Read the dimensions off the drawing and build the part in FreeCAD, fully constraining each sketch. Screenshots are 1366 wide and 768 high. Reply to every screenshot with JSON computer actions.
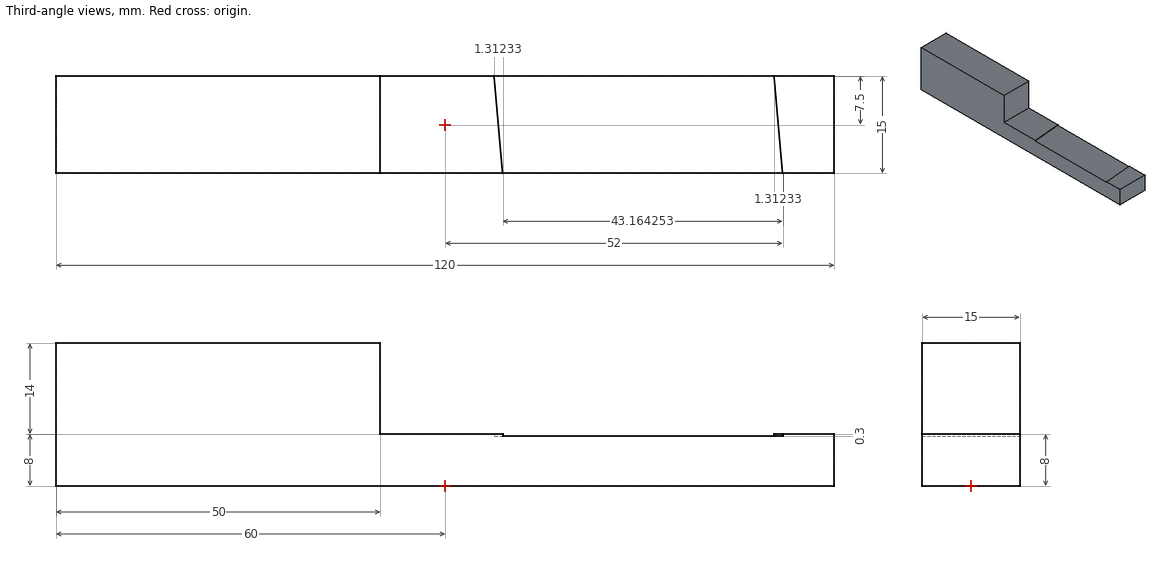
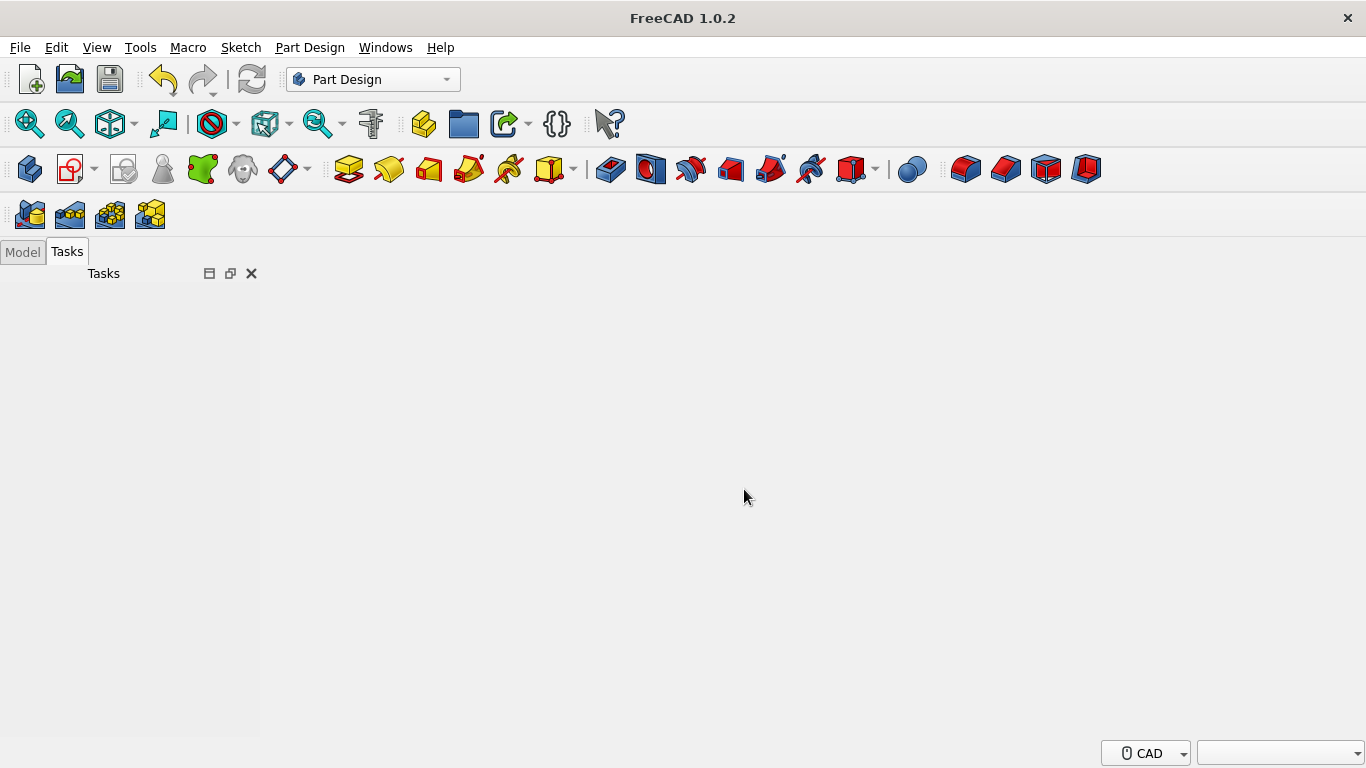
{"action": "left_click", "coordinate": [30, 80]}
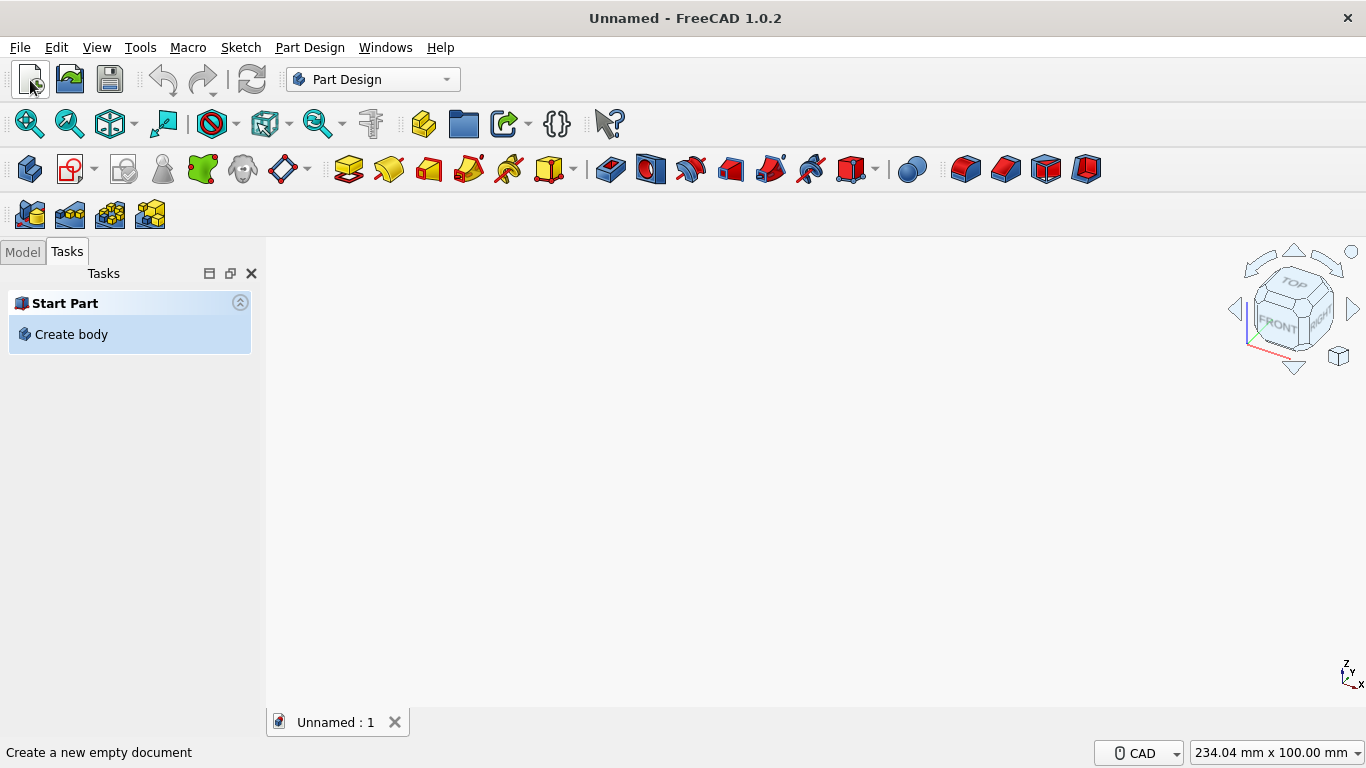
{"action": "left_click", "coordinate": [70, 170]}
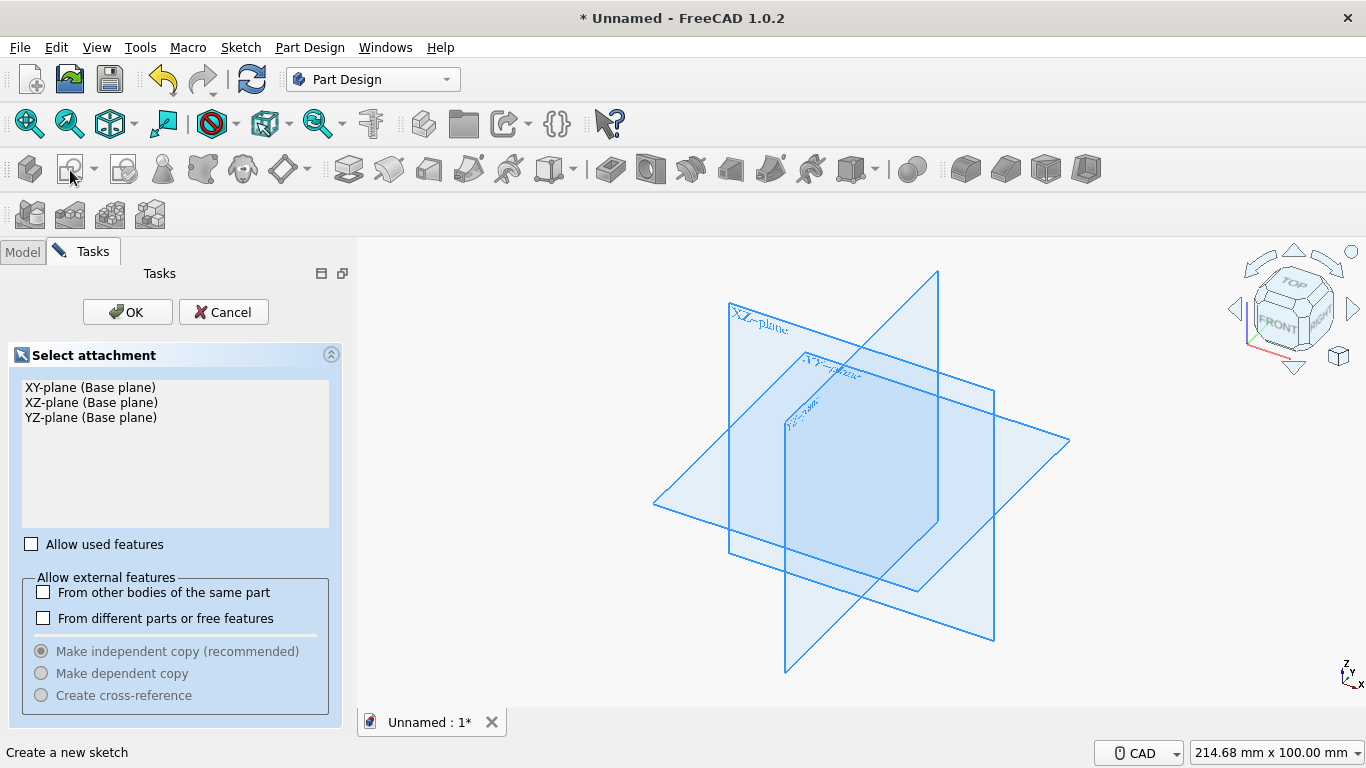
{"action": "left_click", "coordinate": [82, 388]}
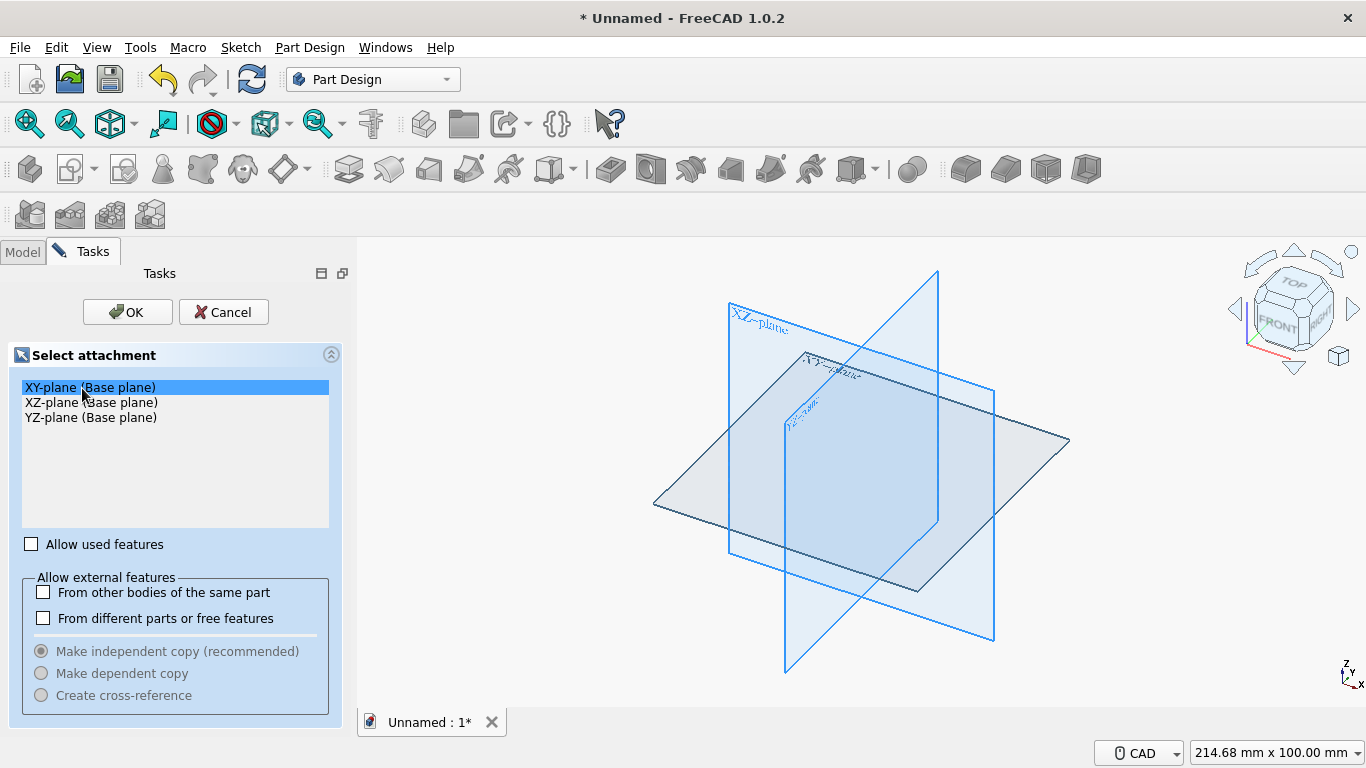
{"action": "left_click", "coordinate": [128, 312]}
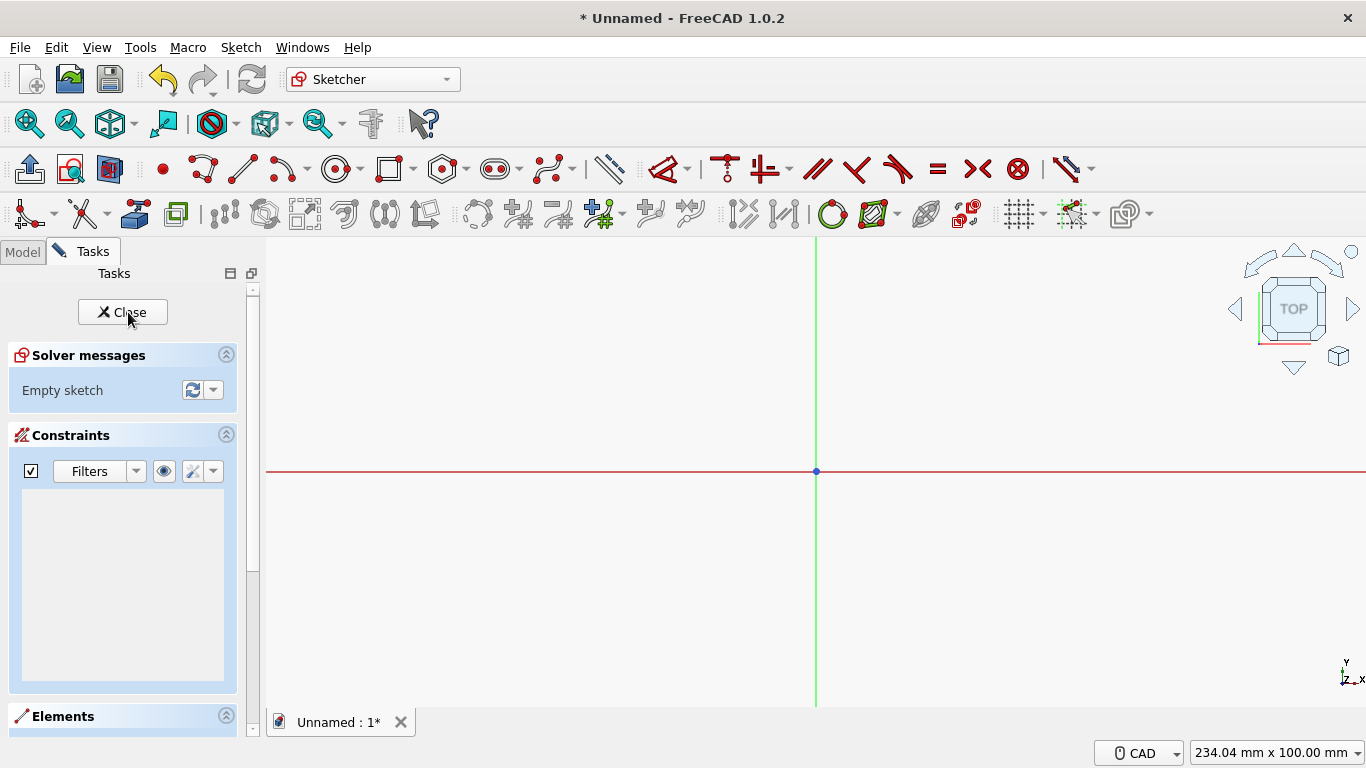
{"action": "left_click", "coordinate": [416, 170]}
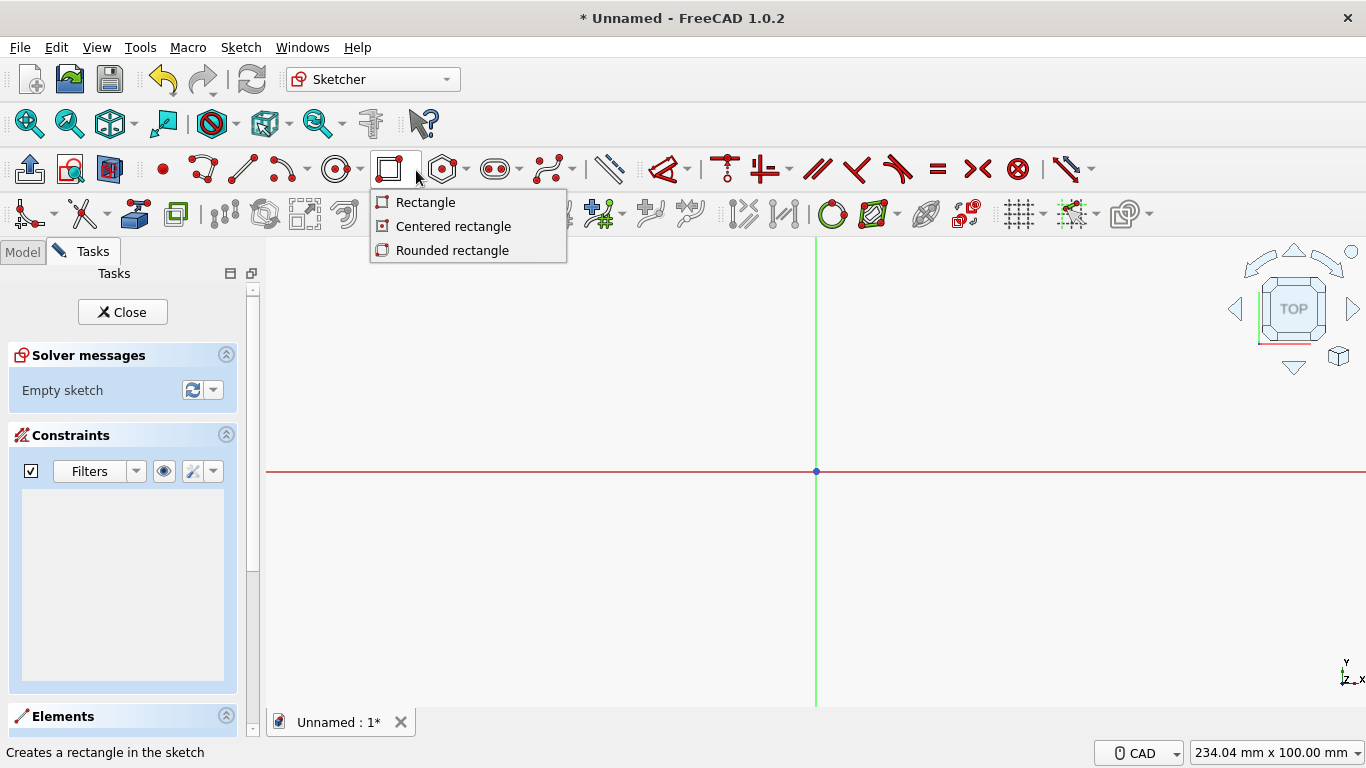
{"action": "left_click", "coordinate": [468, 226]}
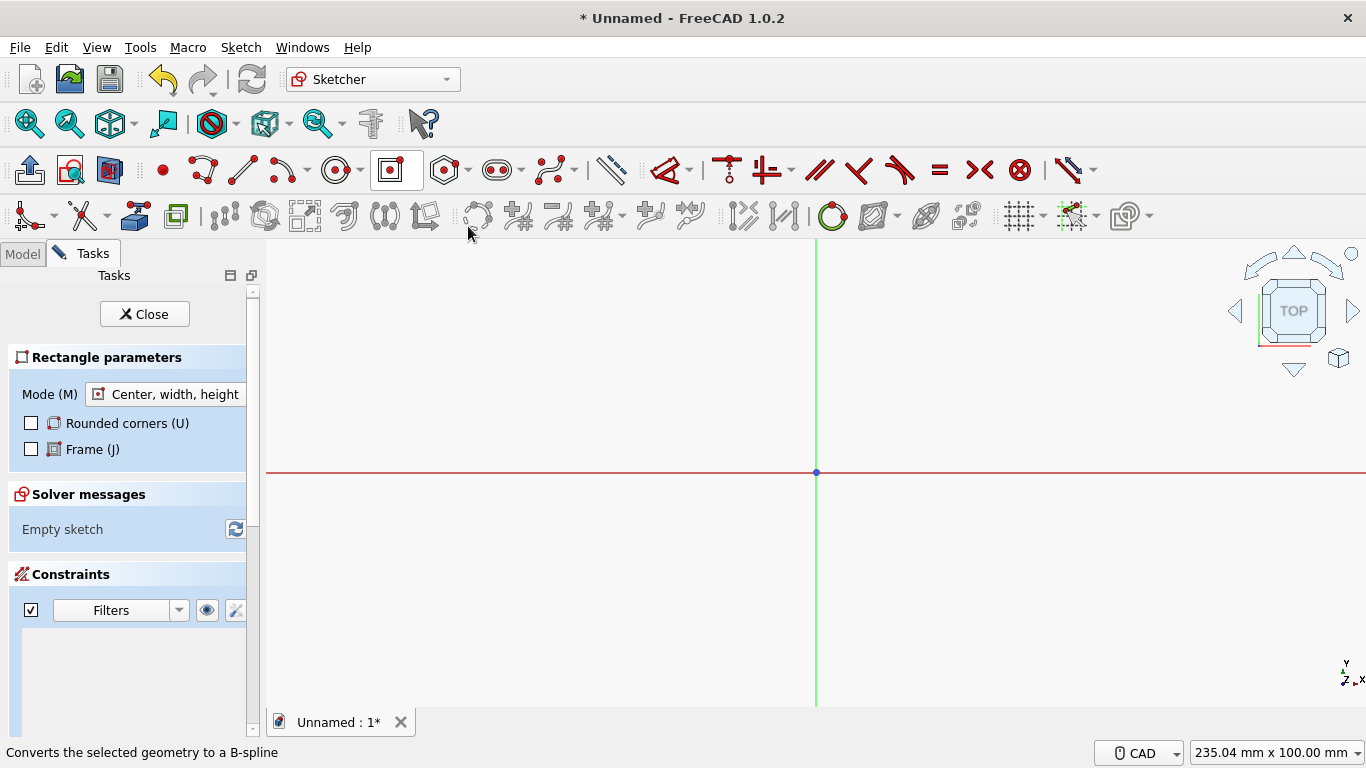
{"action": "left_click", "coordinate": [816, 473]}
{"action": "mouse_move", "coordinate": [1097, 438]}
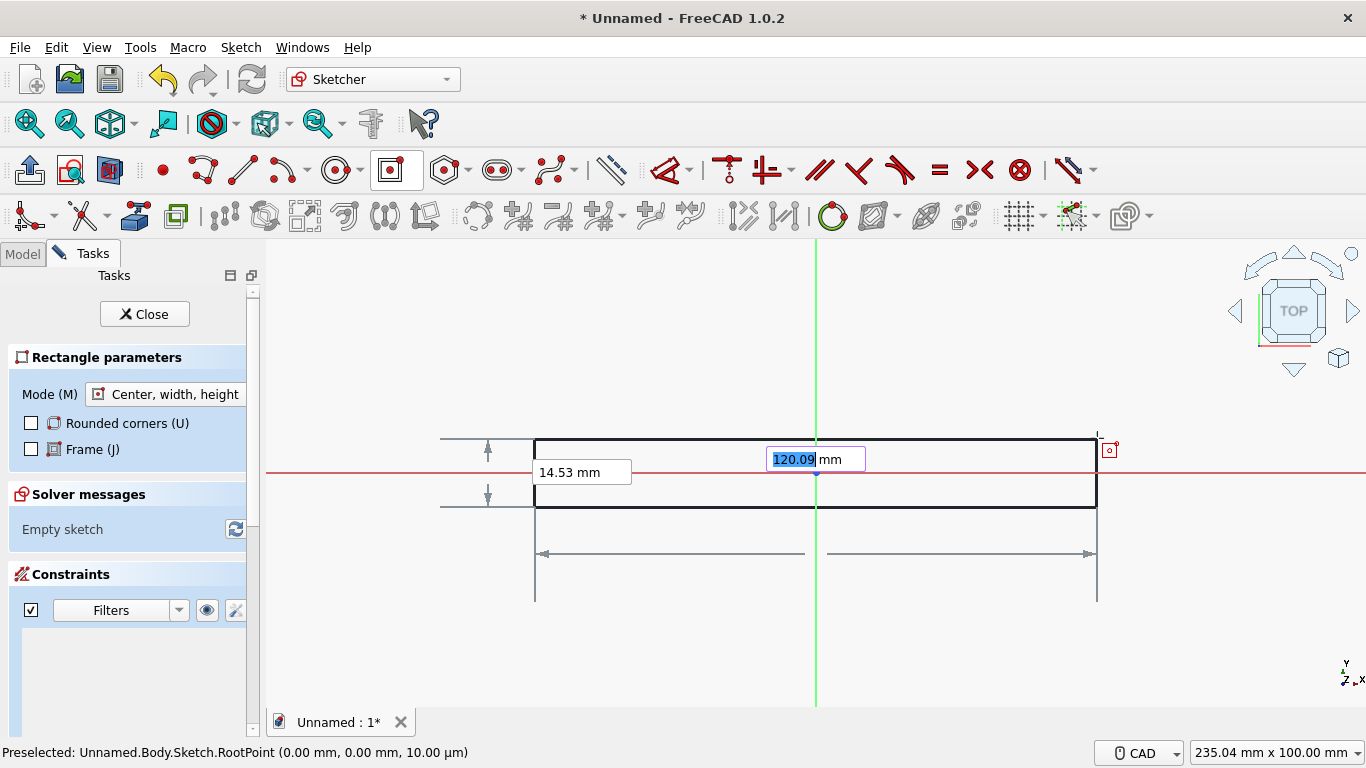
{"action": "type", "text": "120"}
{"action": "key", "text": "Tab"}
{"action": "type", "text": "15"}
{"action": "key", "text": "Return"}
{"action": "key", "text": "Escape"}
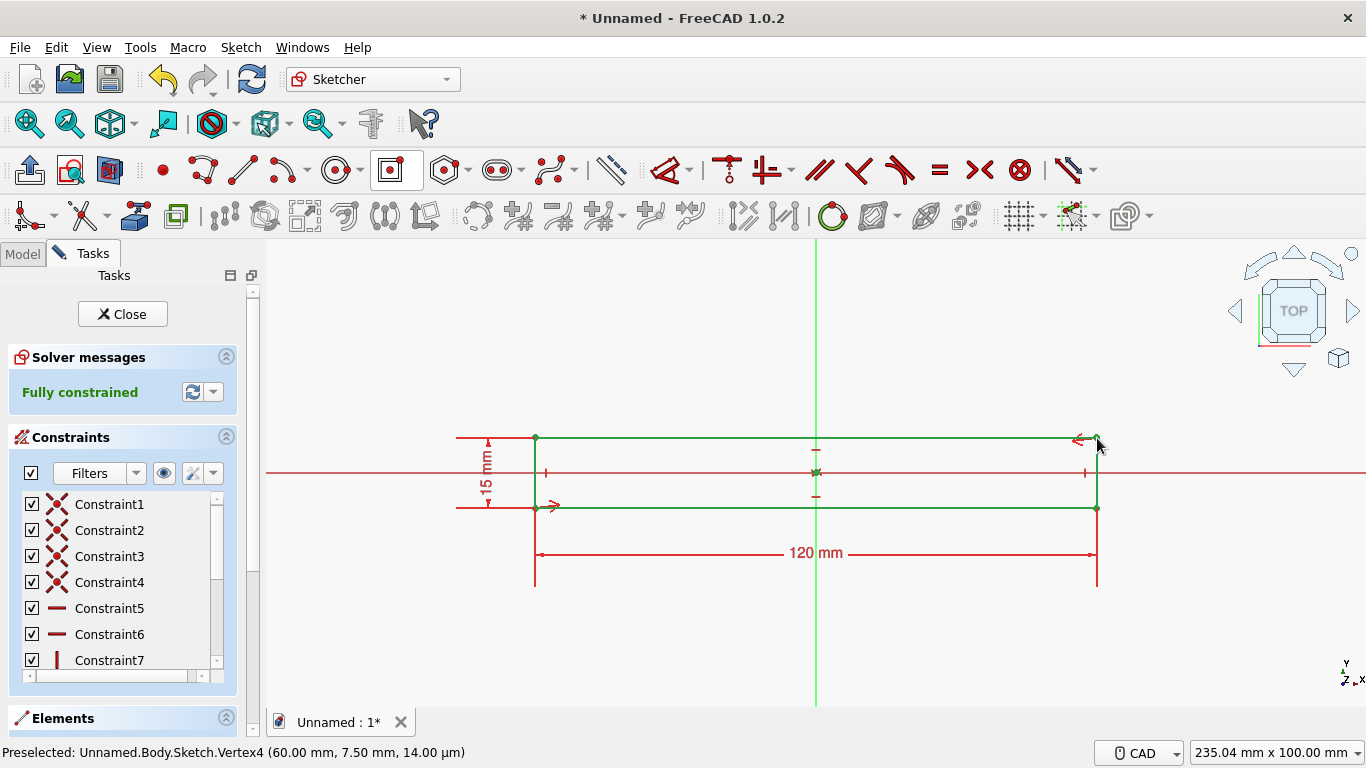
{"action": "left_click", "coordinate": [123, 314]}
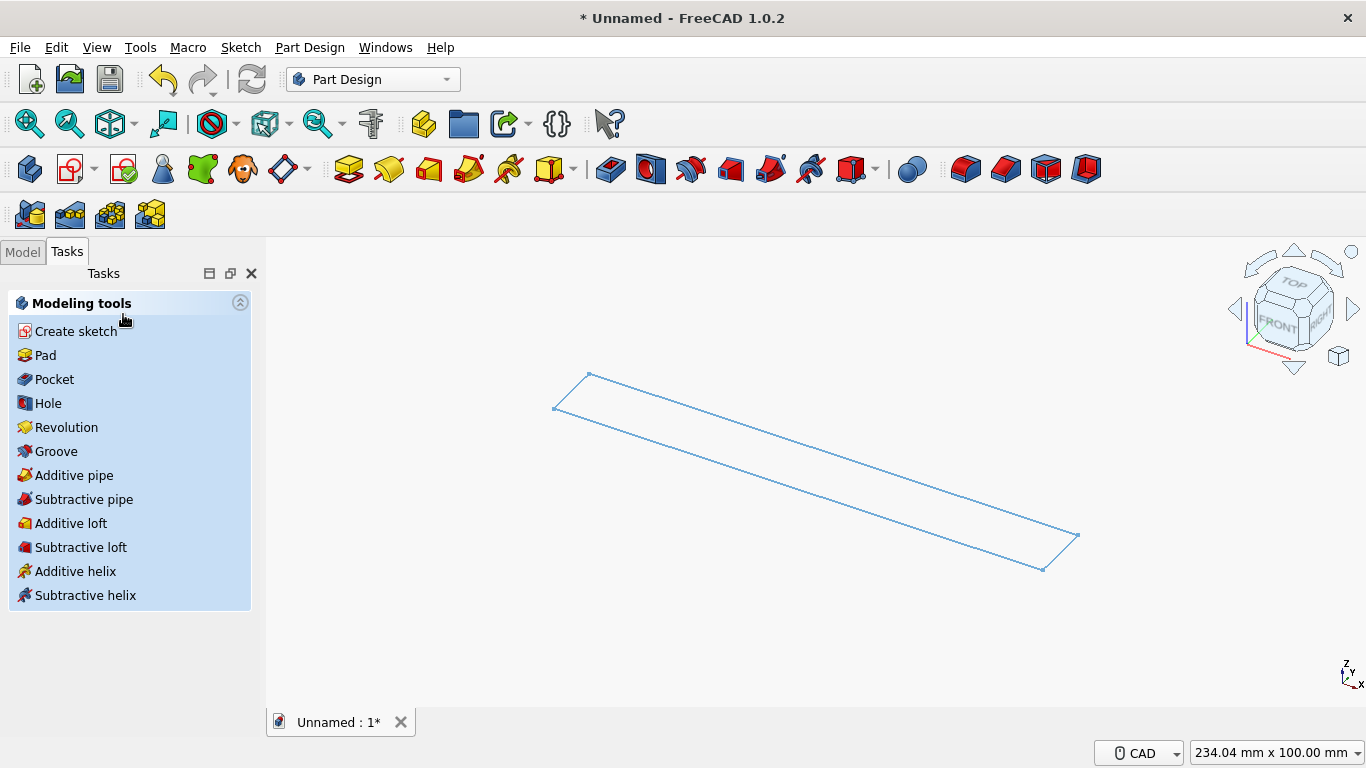
{"action": "left_click", "coordinate": [350, 170]}